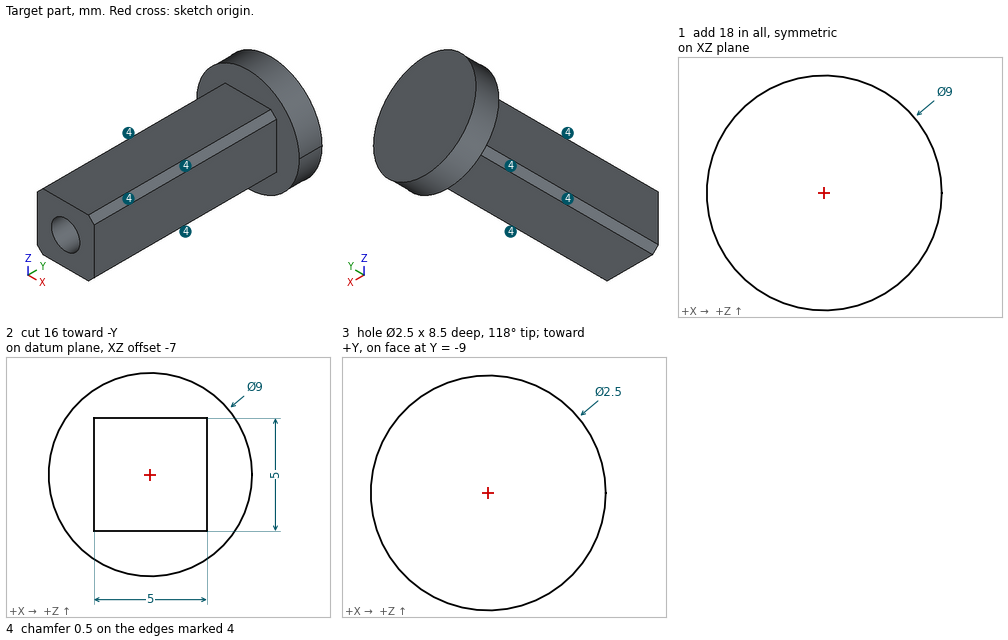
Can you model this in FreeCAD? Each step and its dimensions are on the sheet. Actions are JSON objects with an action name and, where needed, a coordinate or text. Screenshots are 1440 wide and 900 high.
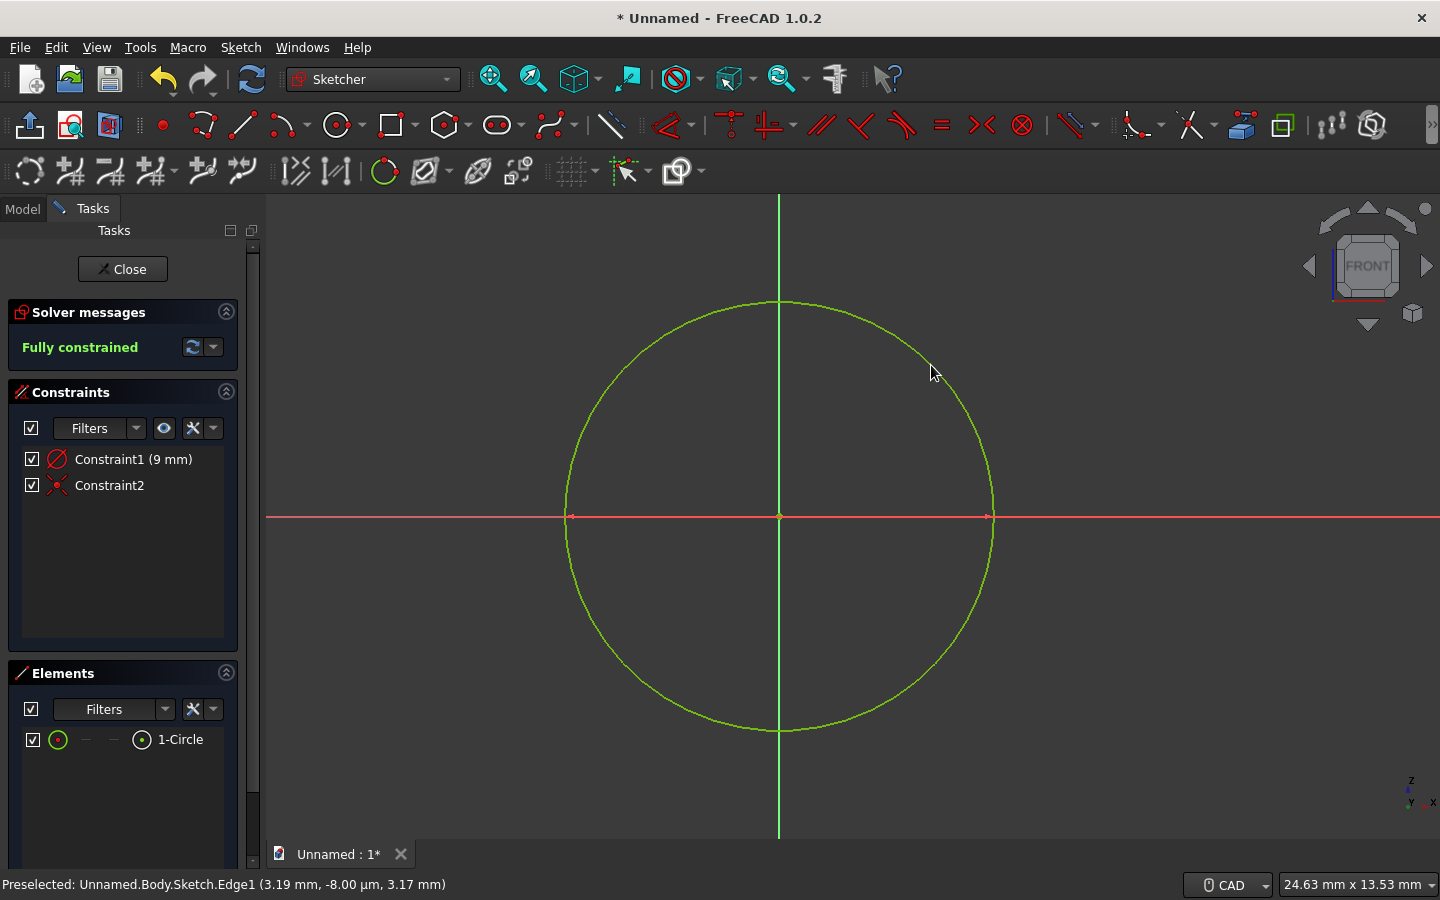
{"action": "left_click", "coordinate": [123, 269]}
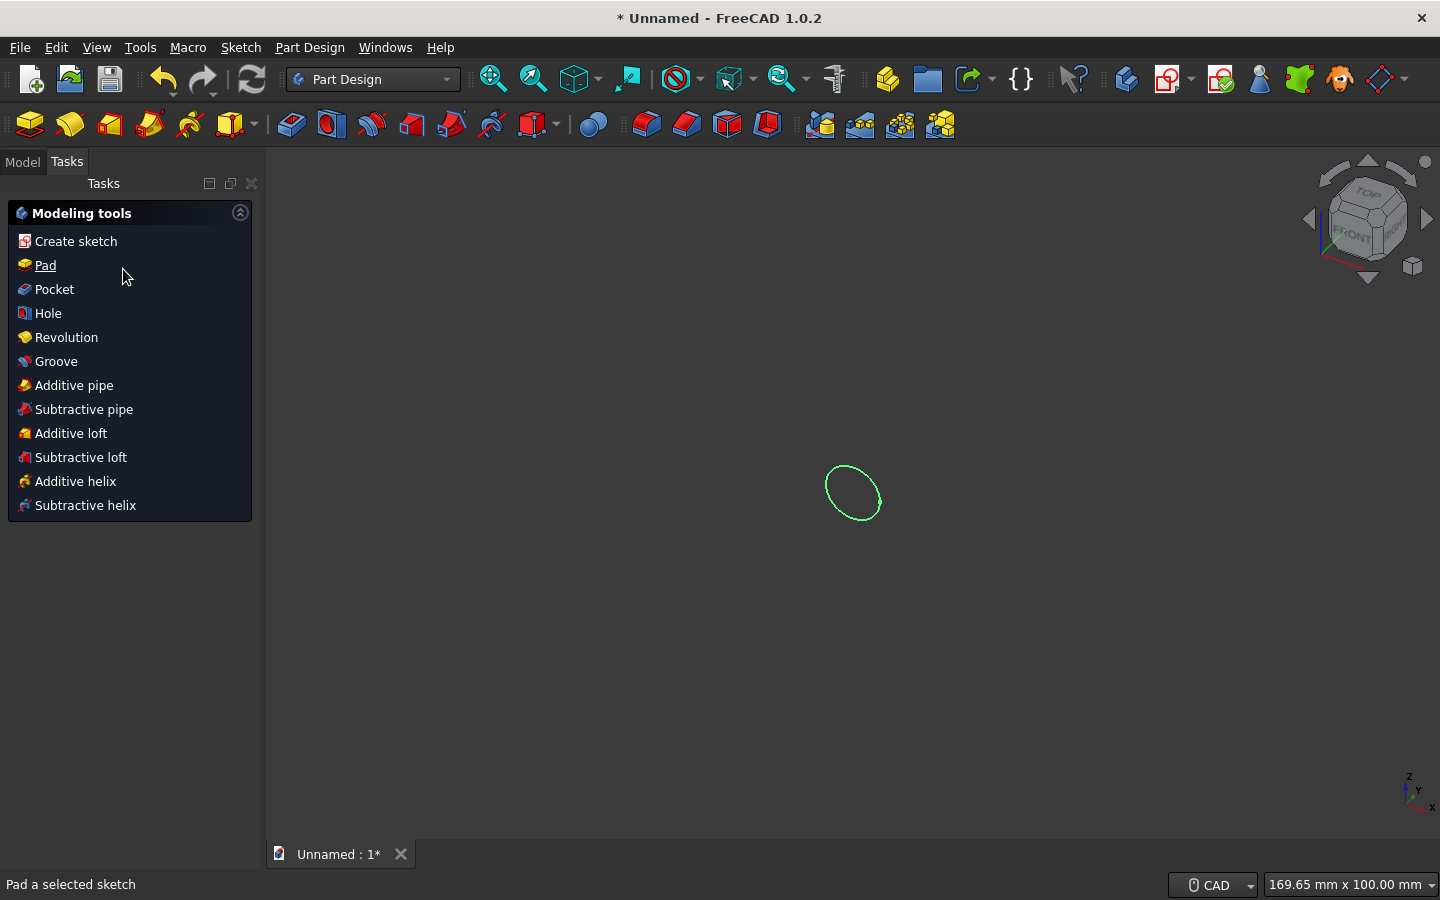
{"action": "left_click", "coordinate": [30, 124]}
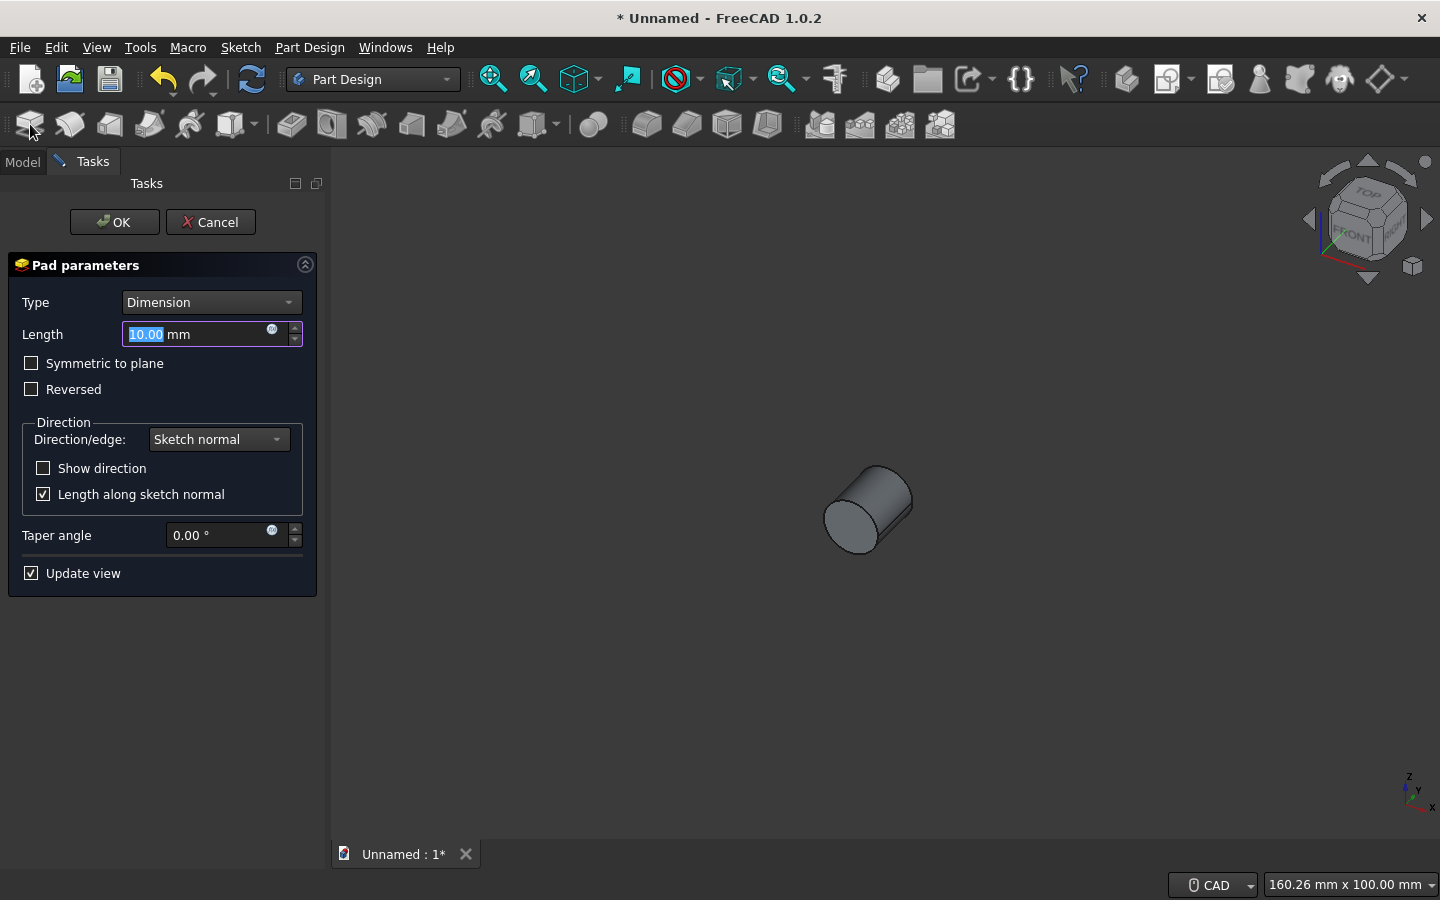
{"action": "type", "text": "18"}
{"action": "key", "text": "Tab"}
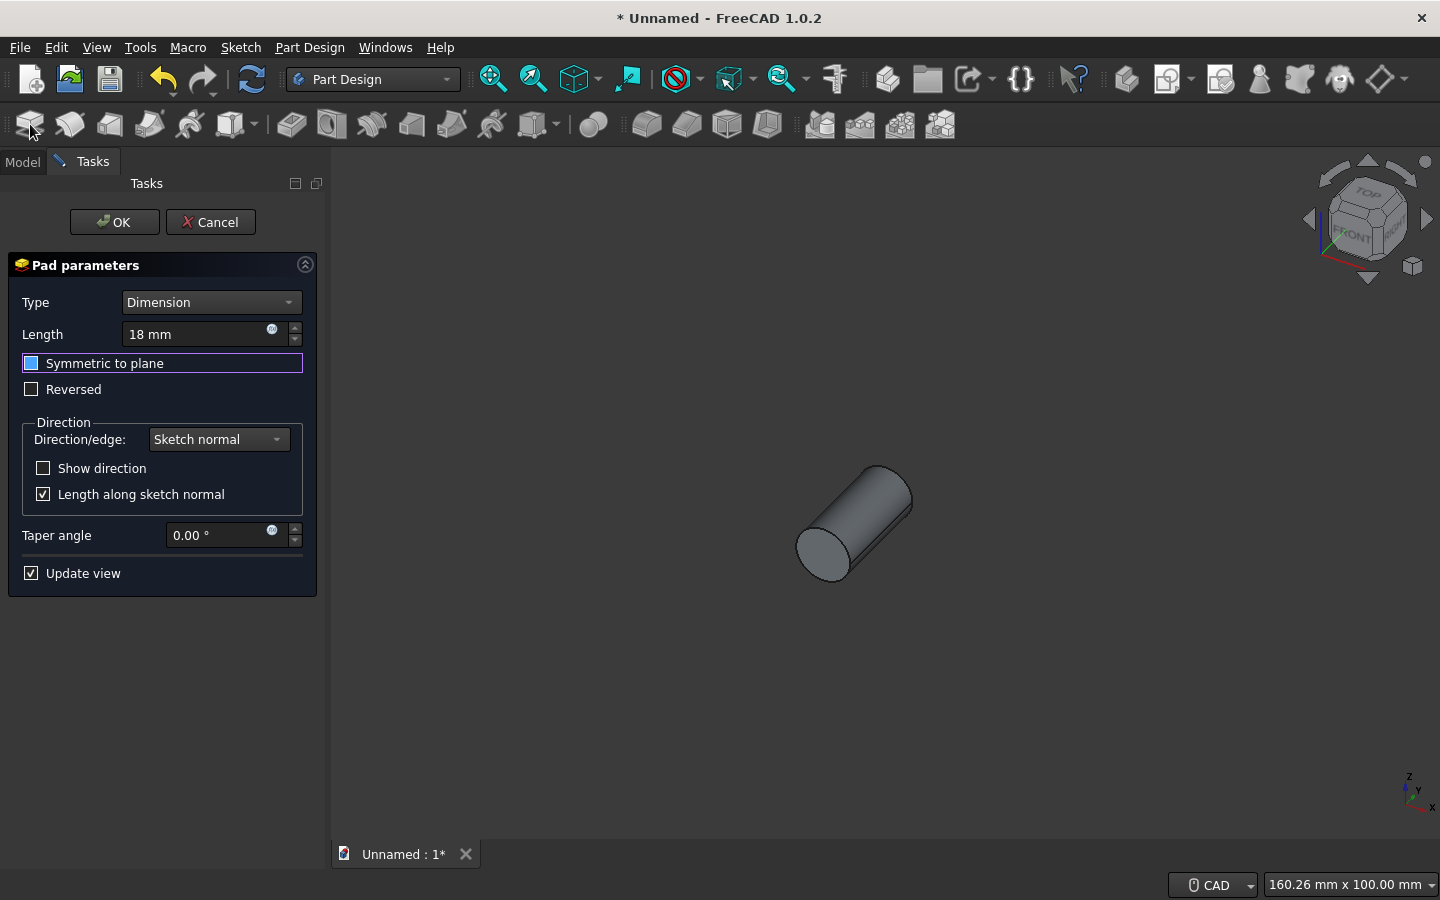
{"action": "left_click", "coordinate": [30, 363]}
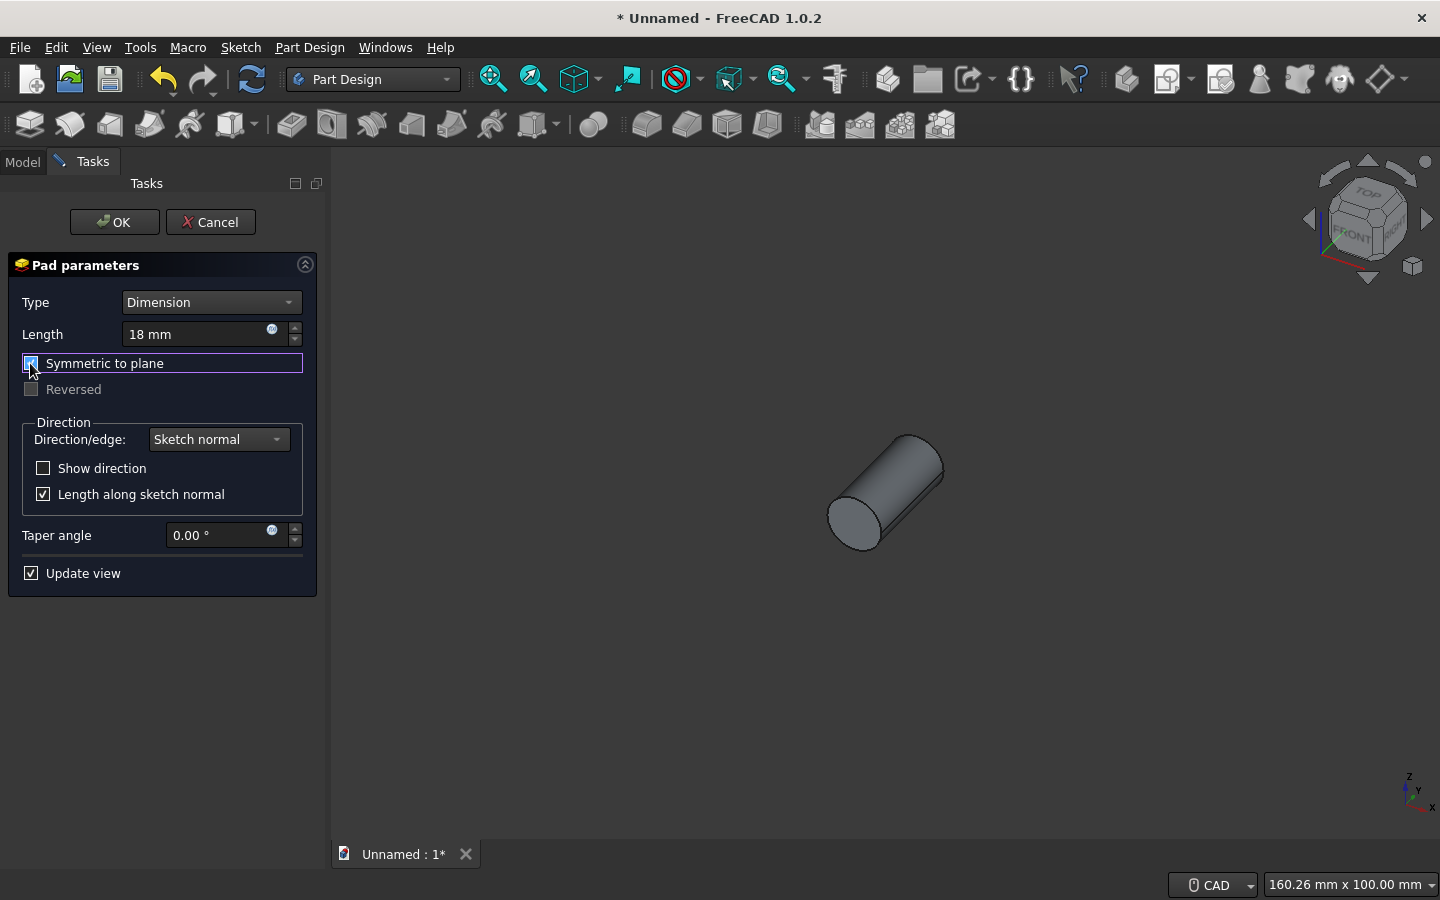
{"action": "left_click", "coordinate": [115, 222]}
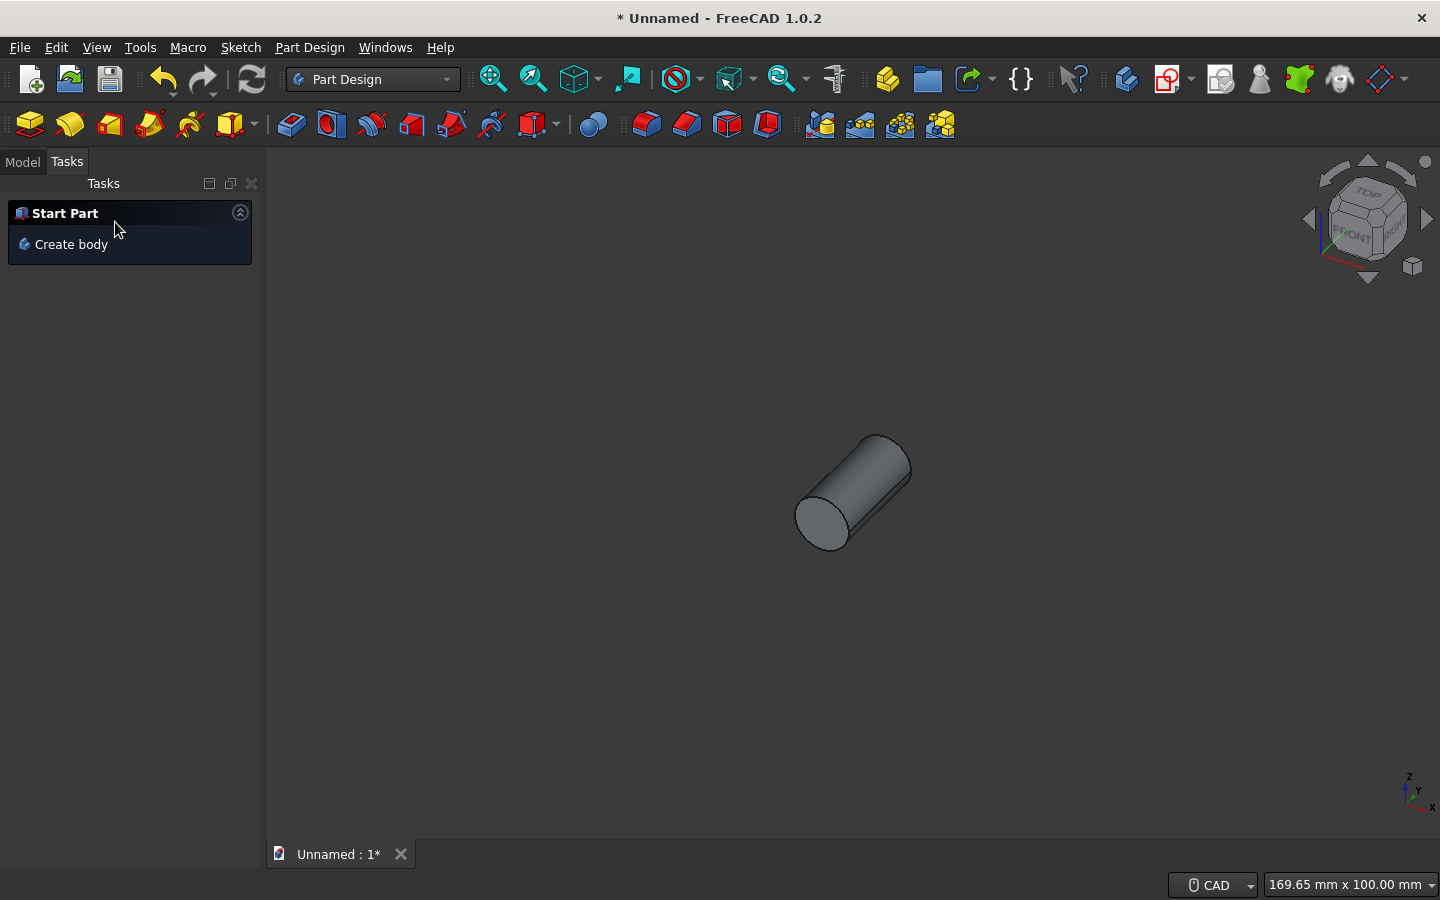
{"action": "left_click", "coordinate": [494, 80]}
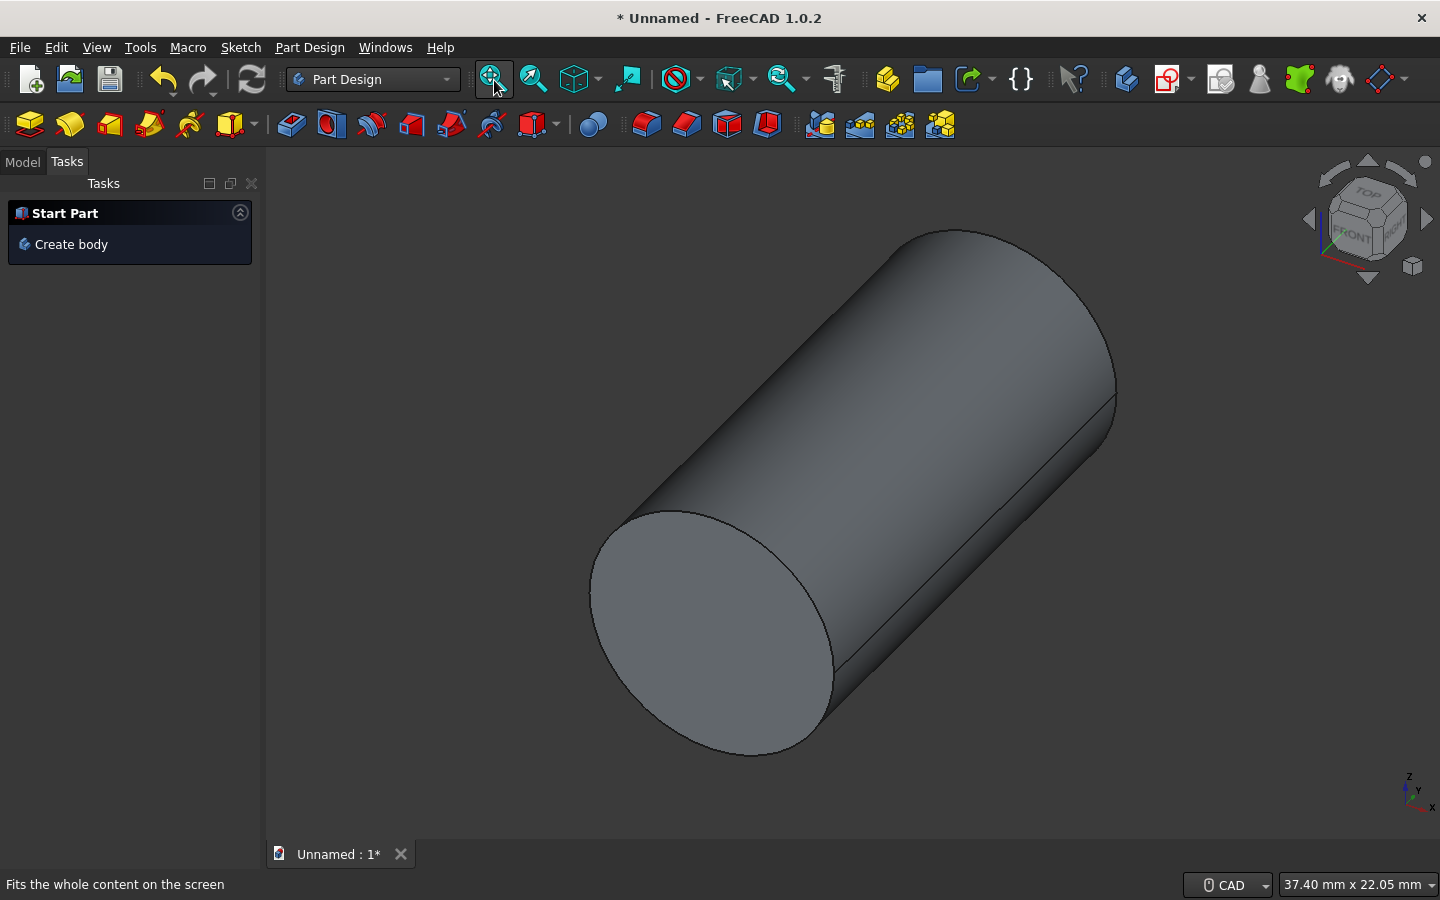
{"action": "left_click", "coordinate": [23, 161]}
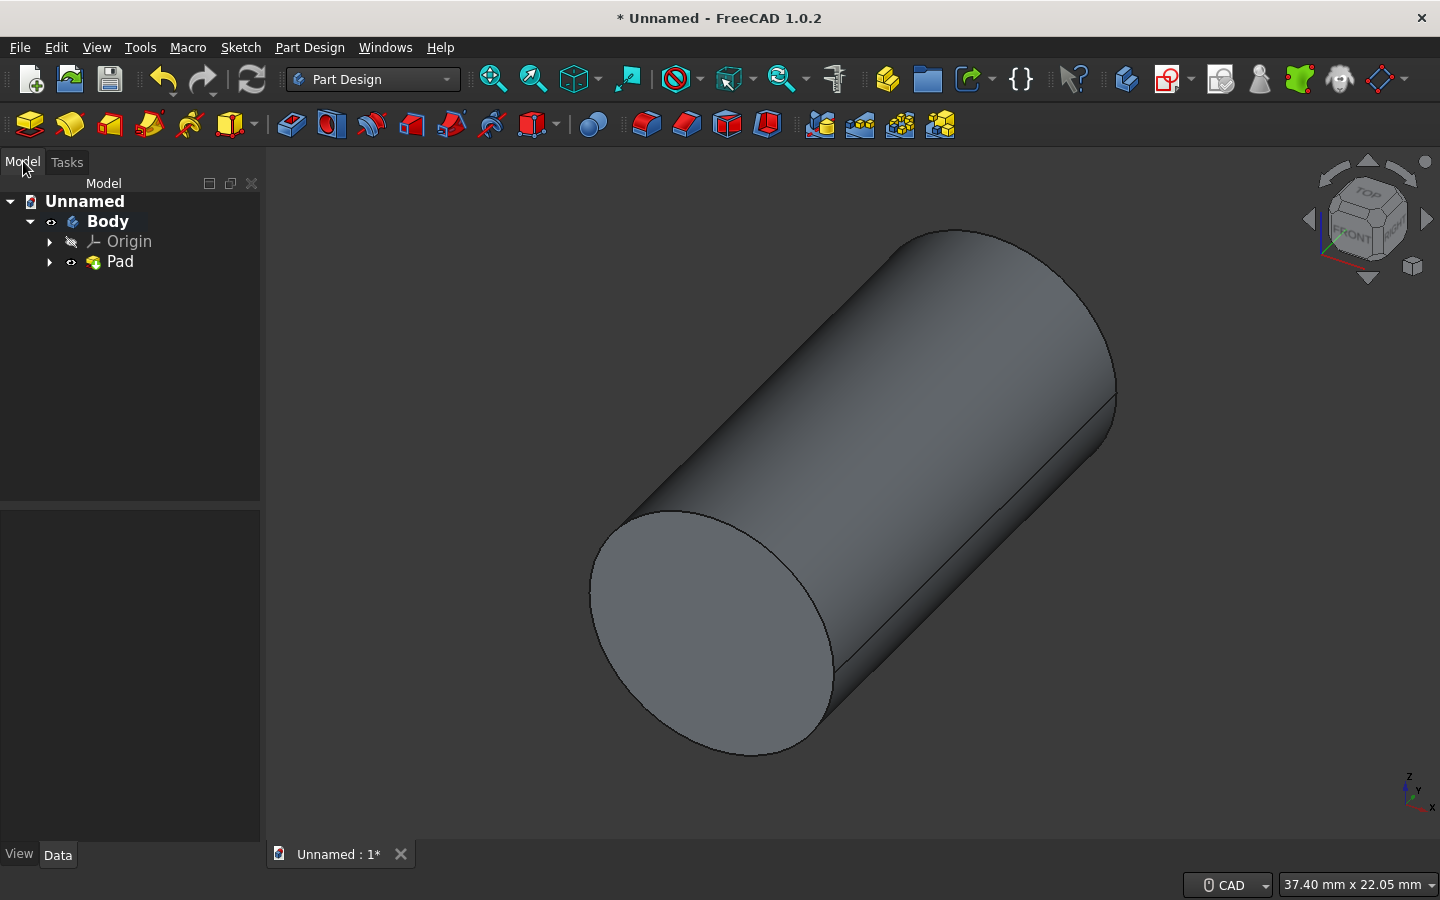
{"action": "left_click", "coordinate": [50, 242]}